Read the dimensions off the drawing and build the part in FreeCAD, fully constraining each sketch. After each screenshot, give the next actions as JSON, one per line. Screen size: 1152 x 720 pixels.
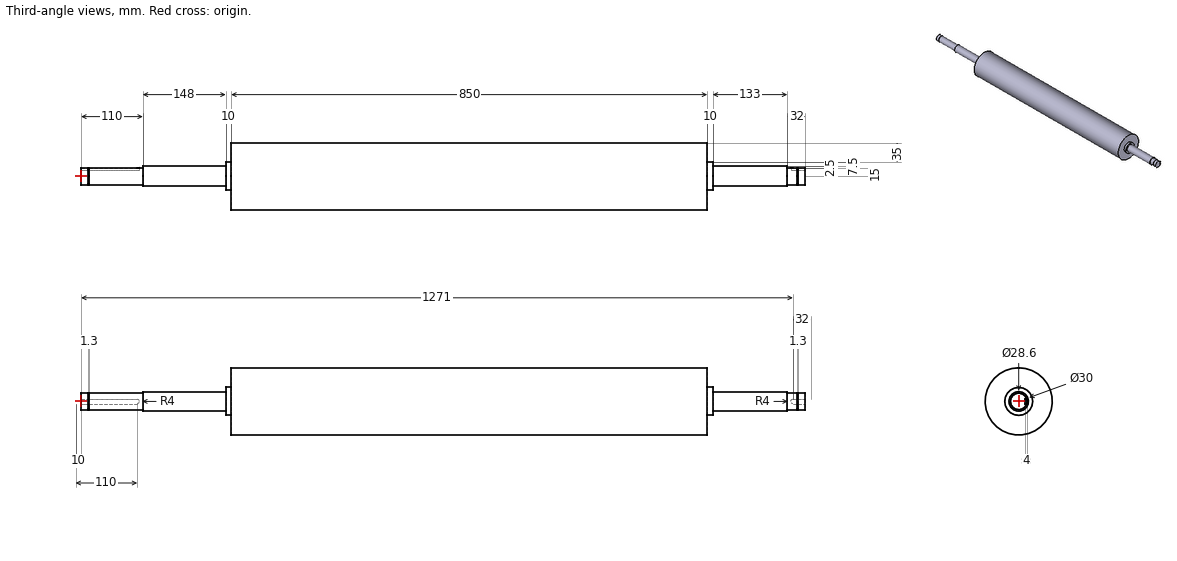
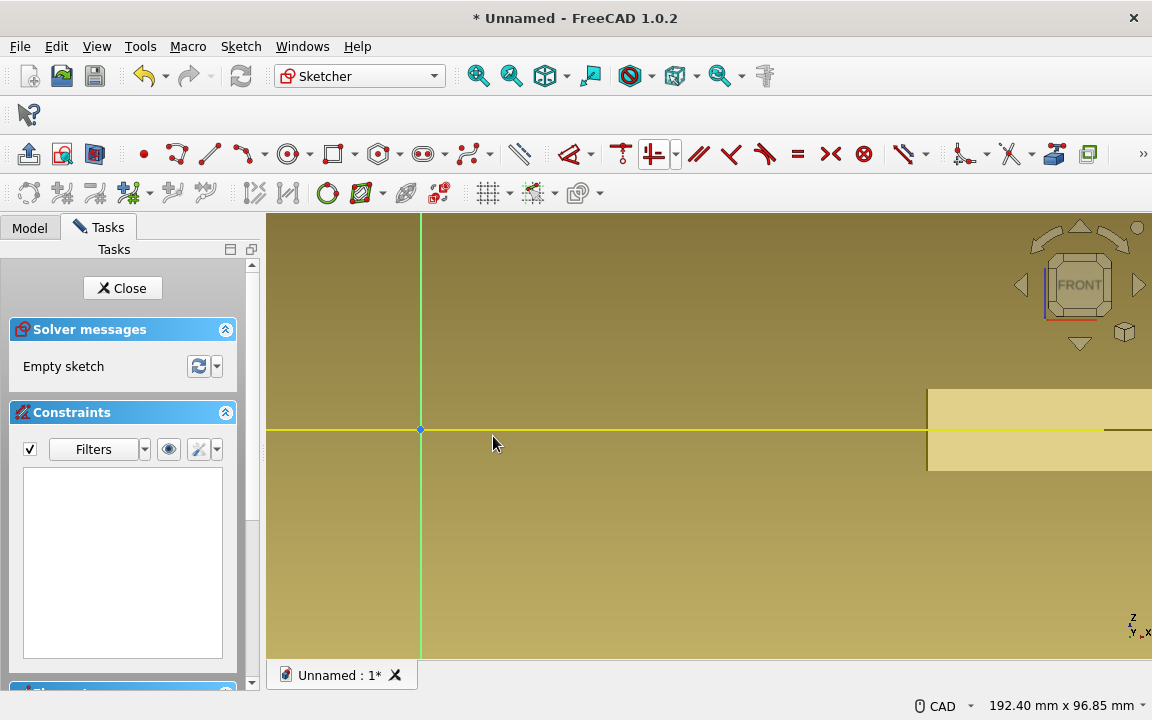
{"action": "key", "text": "g m"}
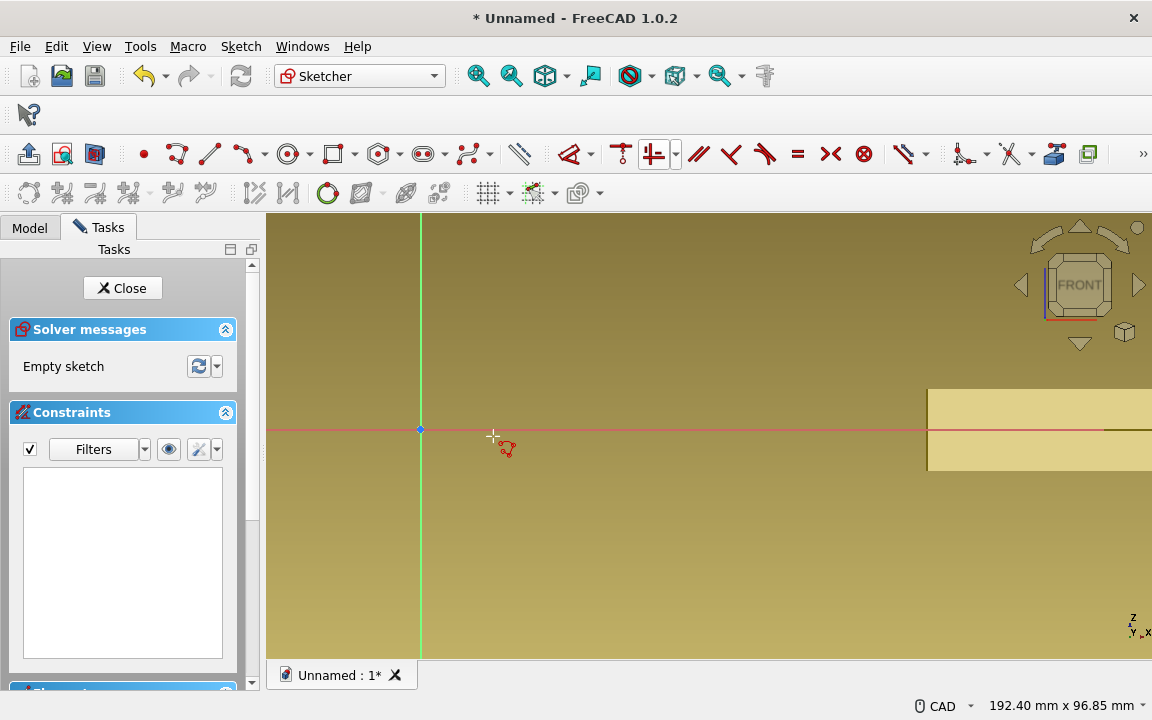
{"action": "left_click", "coordinate": [881, 448]}
{"action": "left_click", "coordinate": [375, 448]}
{"action": "left_click", "coordinate": [375, 411]}
{"action": "left_click", "coordinate": [881, 411]}
{"action": "right_click", "coordinate": [881, 411]}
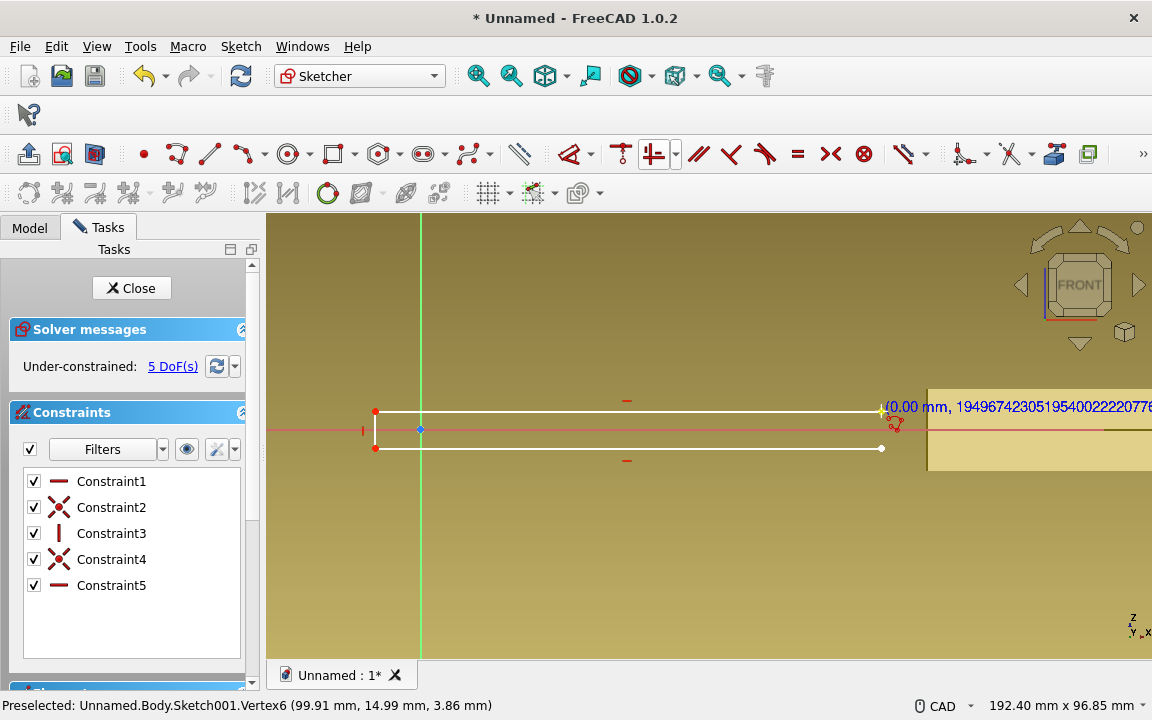
{"action": "key", "text": "g 3 a"}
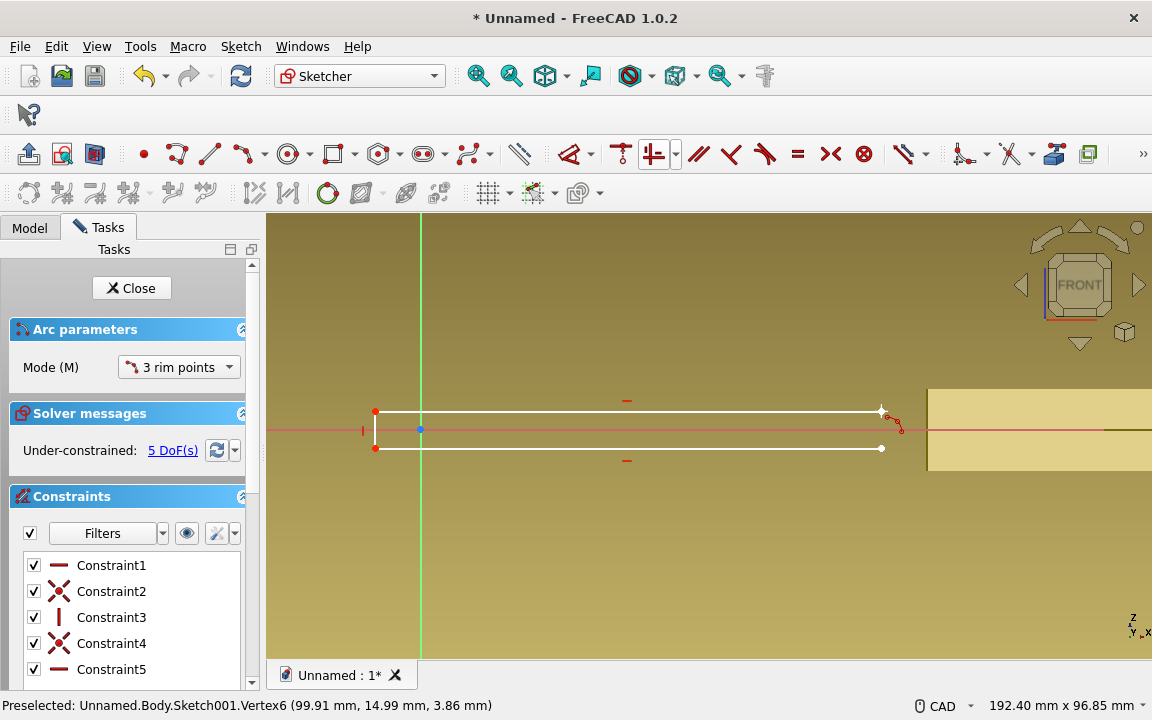
{"action": "left_click", "coordinate": [881, 412]}
{"action": "left_click", "coordinate": [881, 449]}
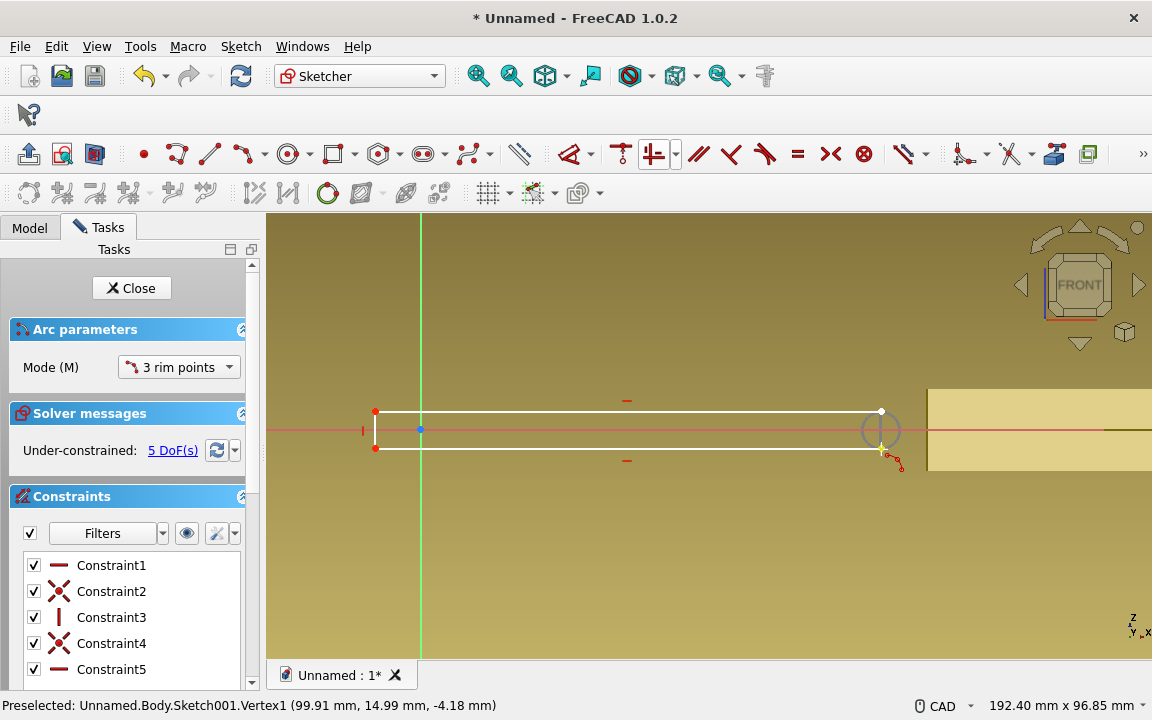
{"action": "scroll", "coordinate": [896, 441], "scroll_direction": "up", "scroll_amount": 2}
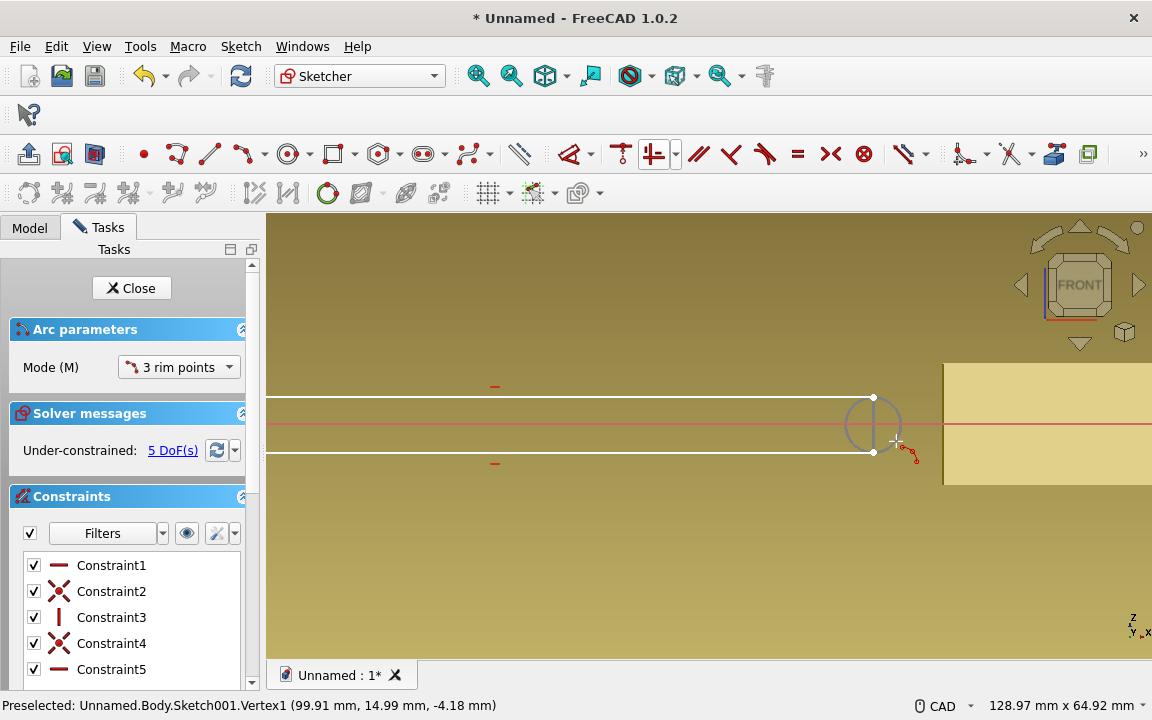
{"action": "left_click", "coordinate": [896, 440]}
{"action": "key", "text": "Escape"}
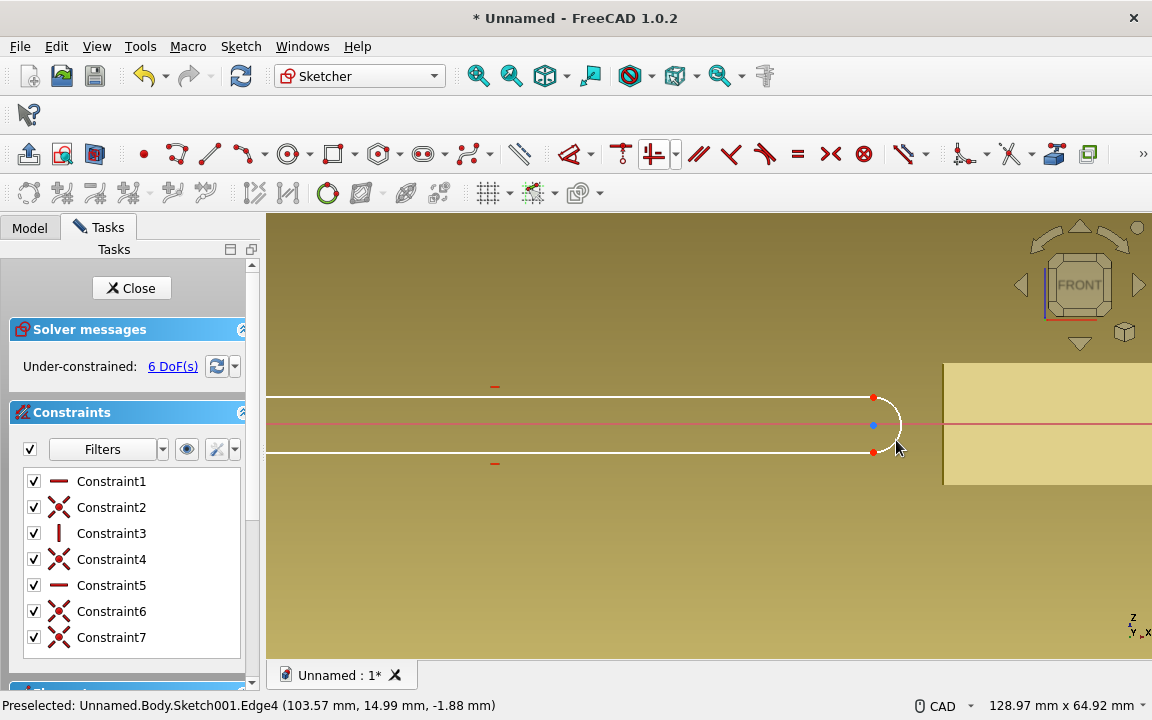
{"action": "left_click", "coordinate": [647, 453]}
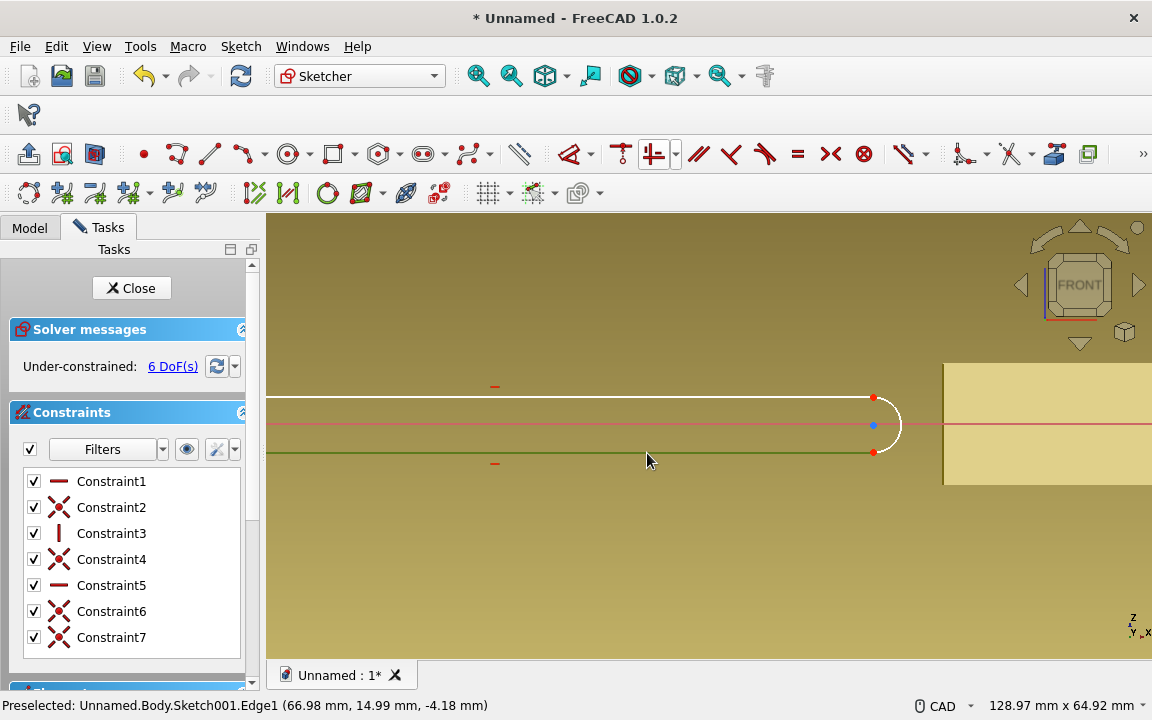
{"action": "left_click", "coordinate": [896, 441]}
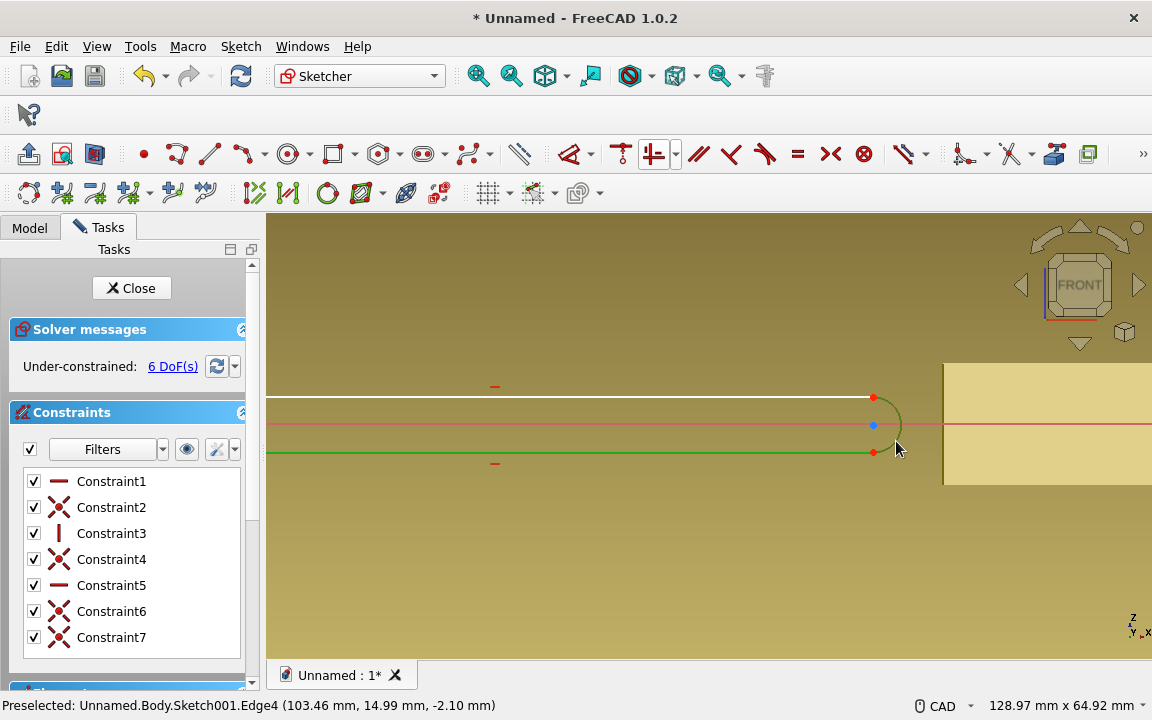
{"action": "key", "text": "t"}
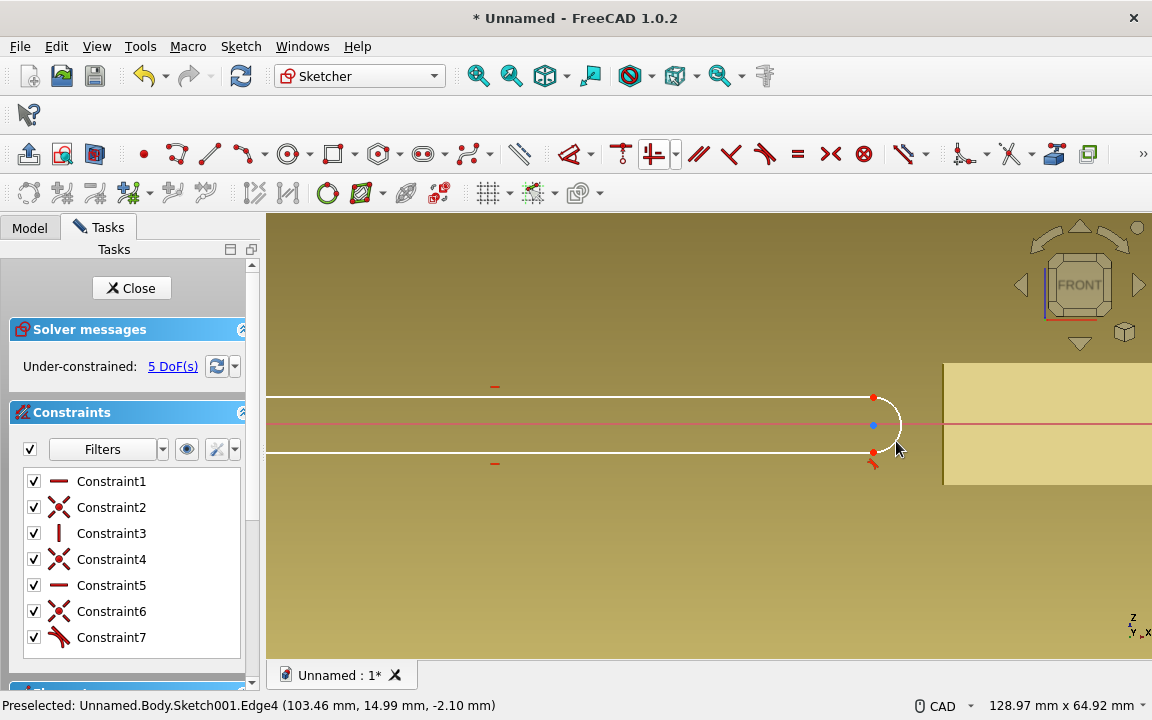
{"action": "left_click", "coordinate": [345, 397]}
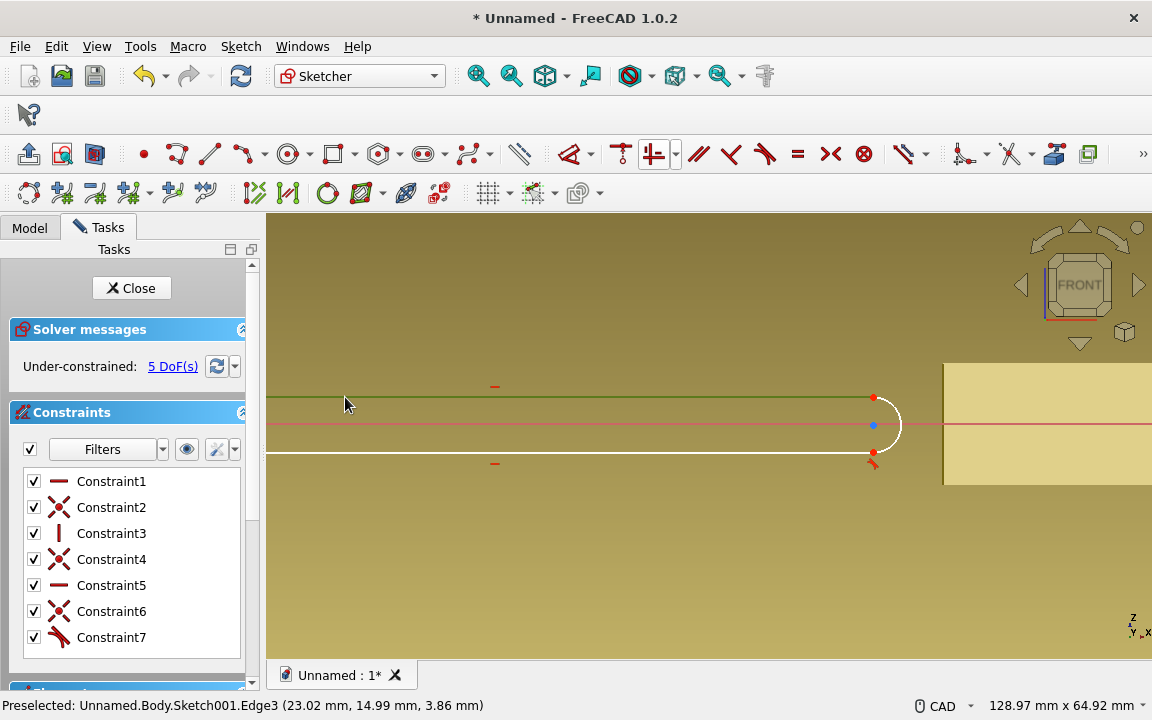
{"action": "left_click", "coordinate": [896, 441]}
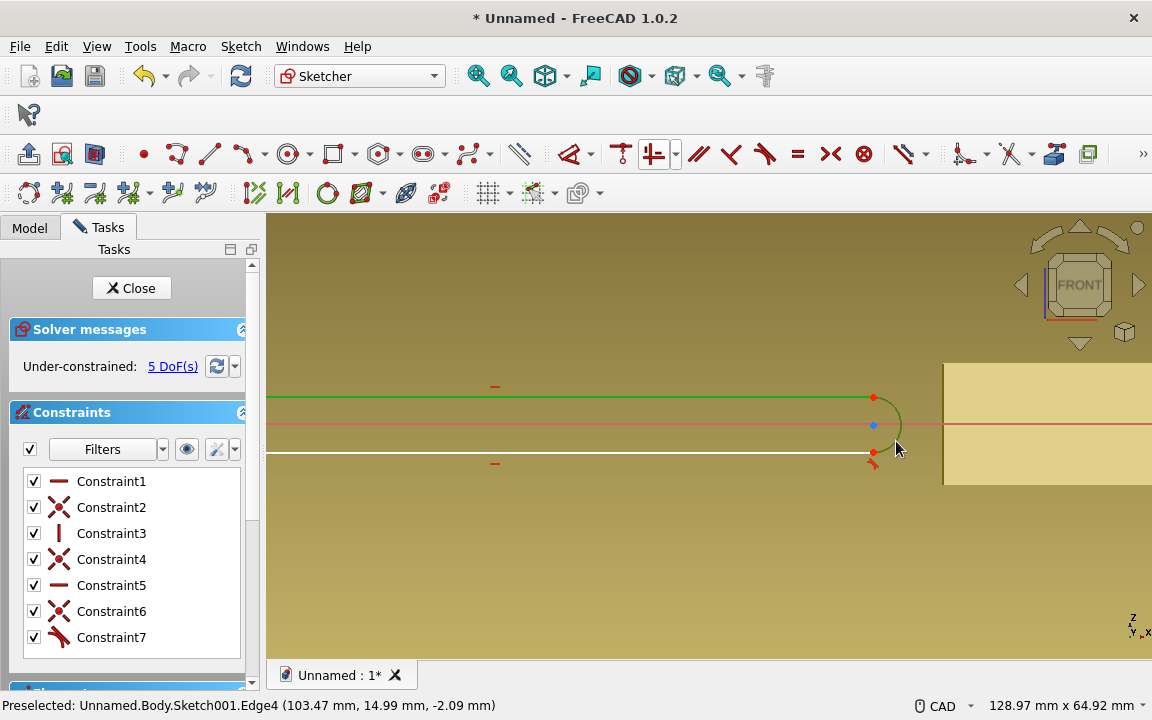
{"action": "left_click", "coordinate": [765, 154]}